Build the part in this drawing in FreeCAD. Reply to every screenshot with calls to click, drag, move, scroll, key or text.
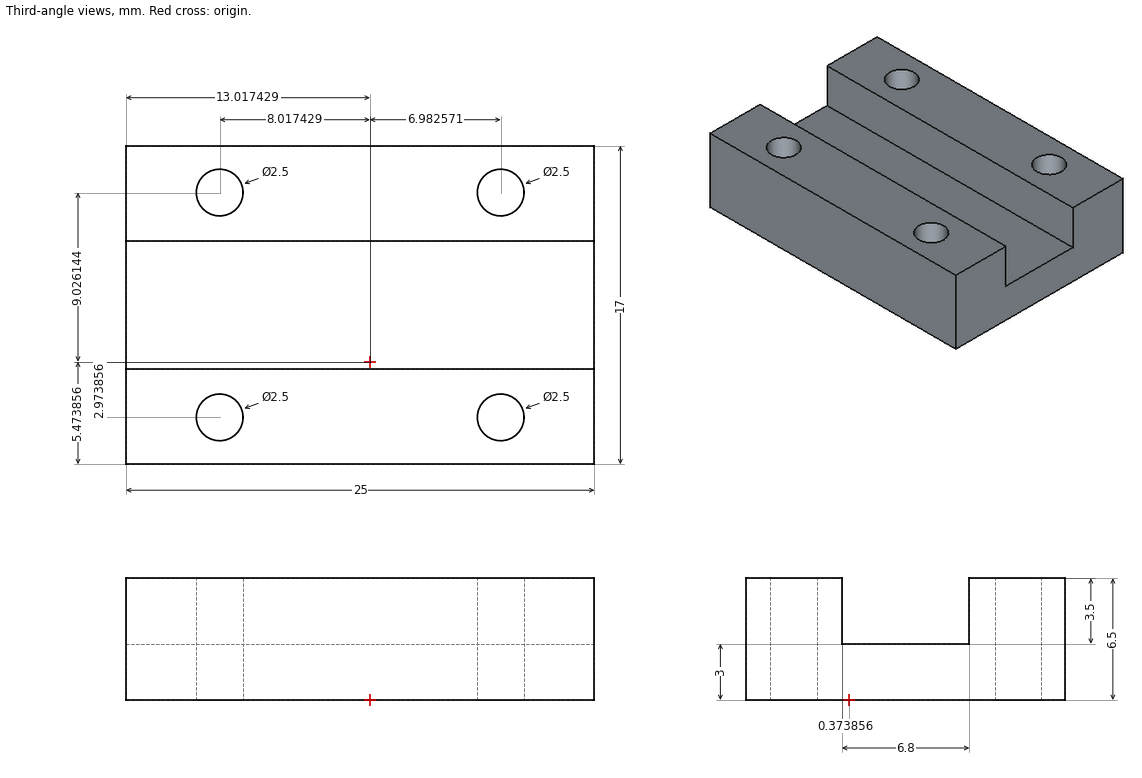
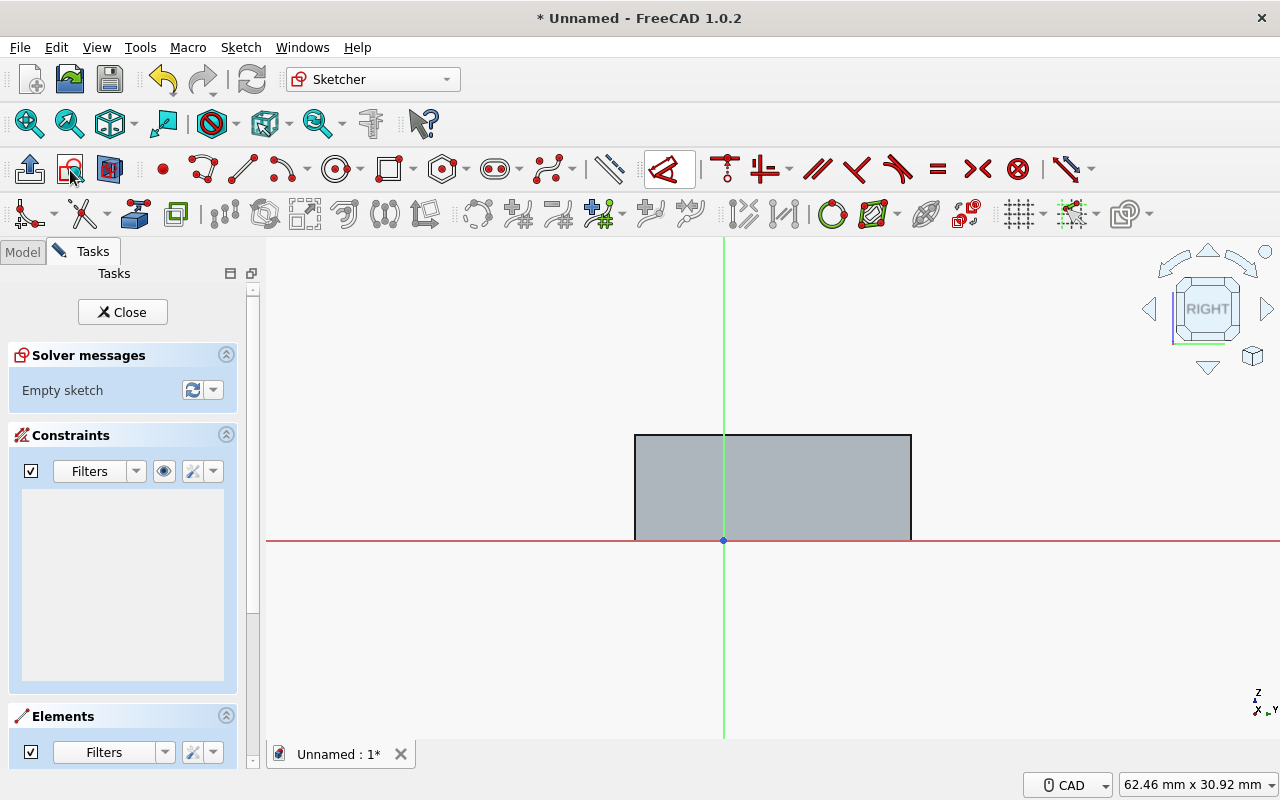
scroll(813, 488, up, 5)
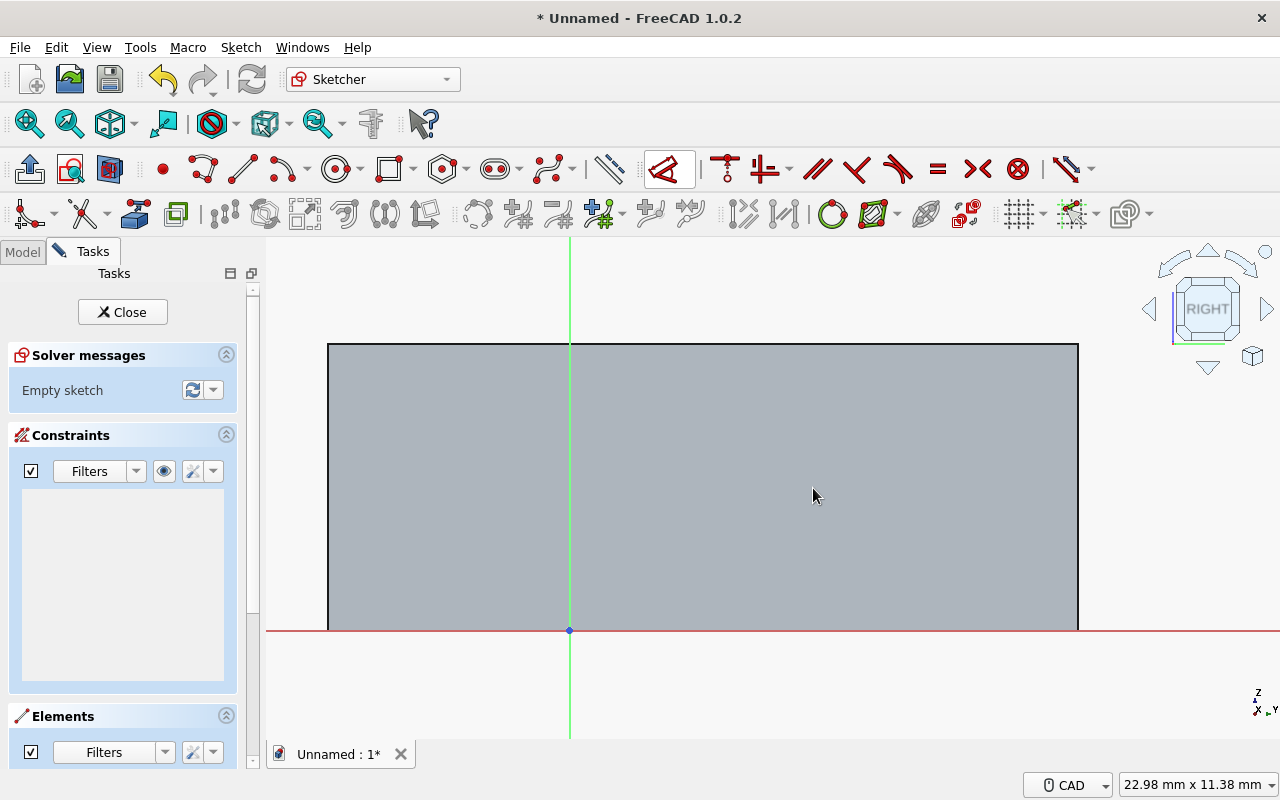
click(390, 170)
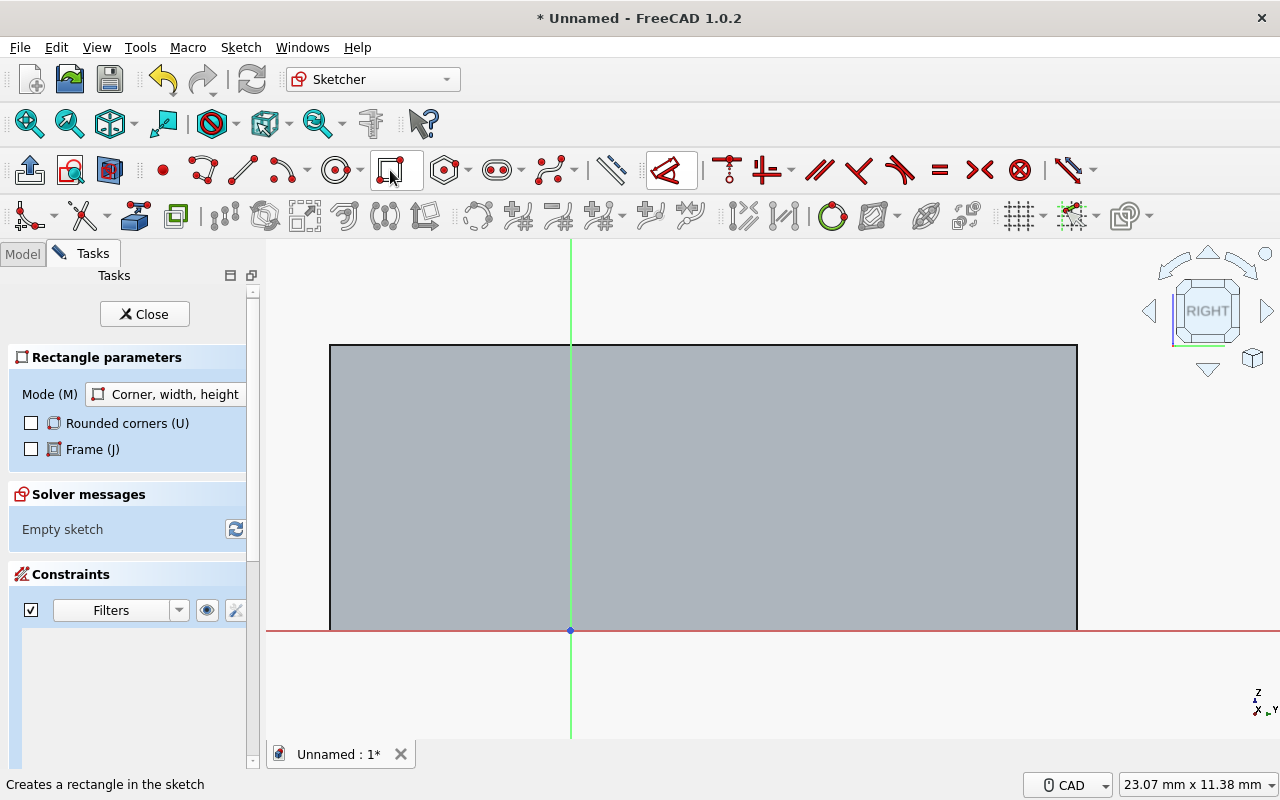
click(554, 345)
move(853, 499)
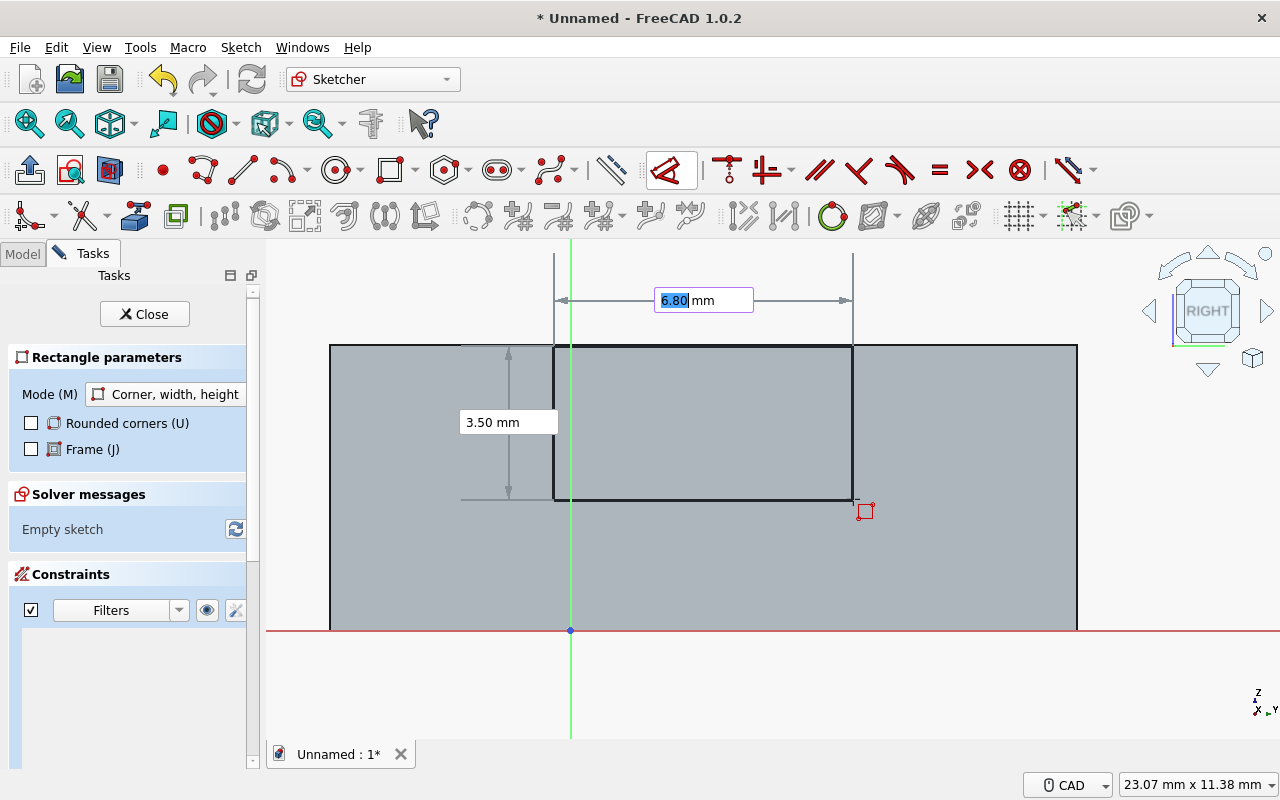
text(6.8)
key(Tab)
text(3.5)
key(Return)
key(Escape)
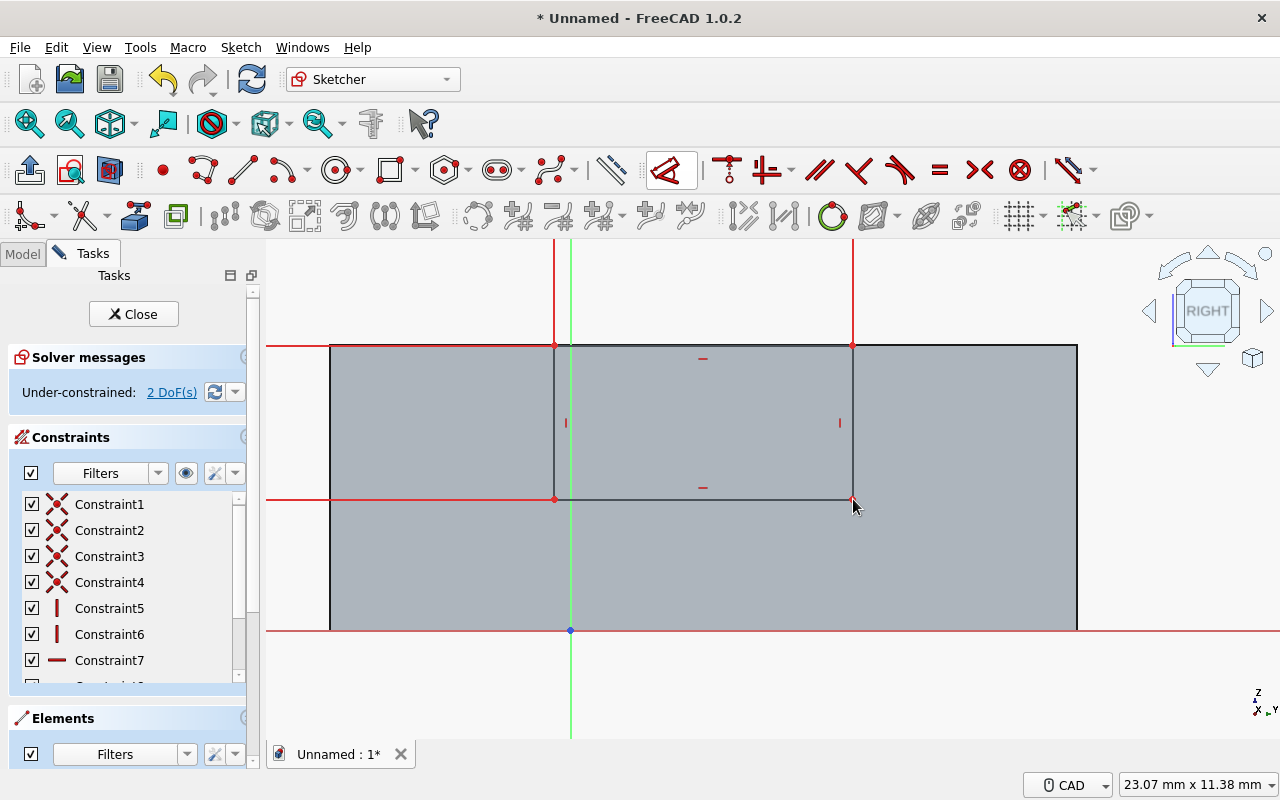
click(666, 170)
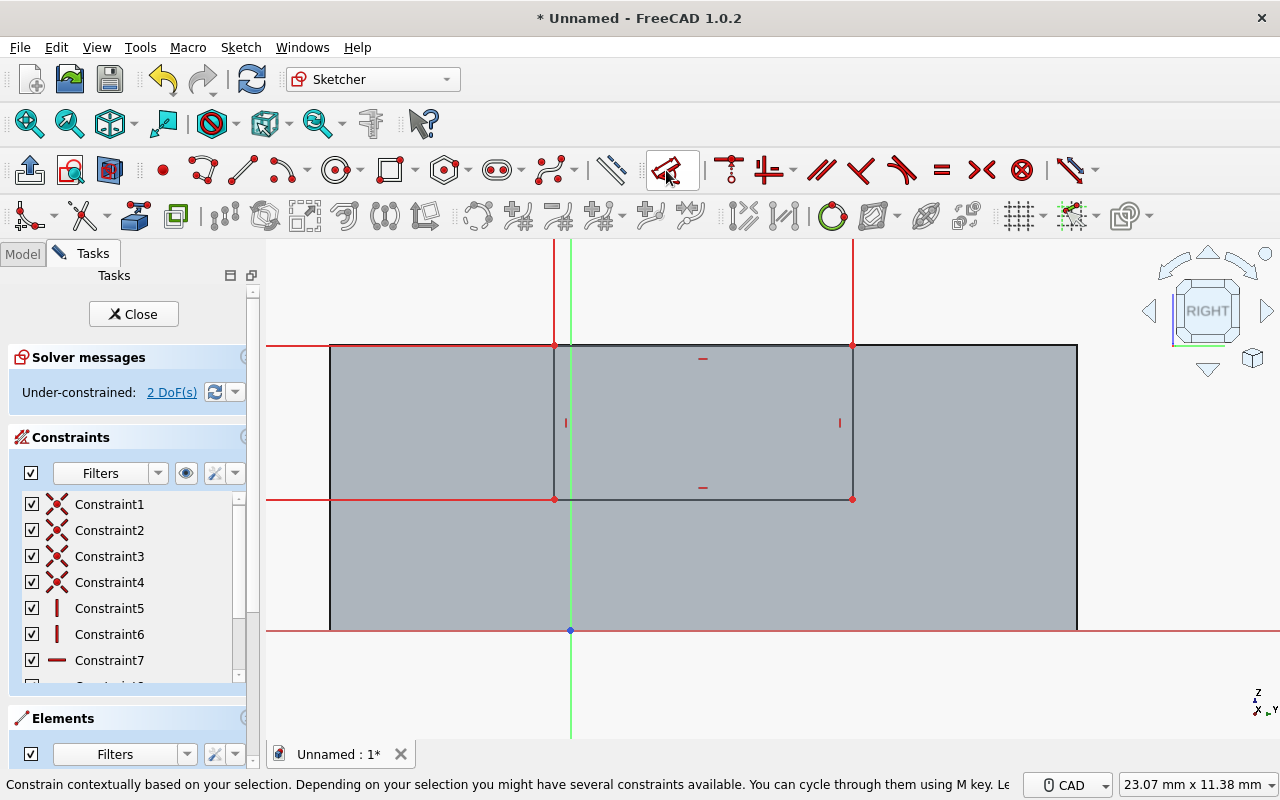
click(554, 500)
click(520, 565)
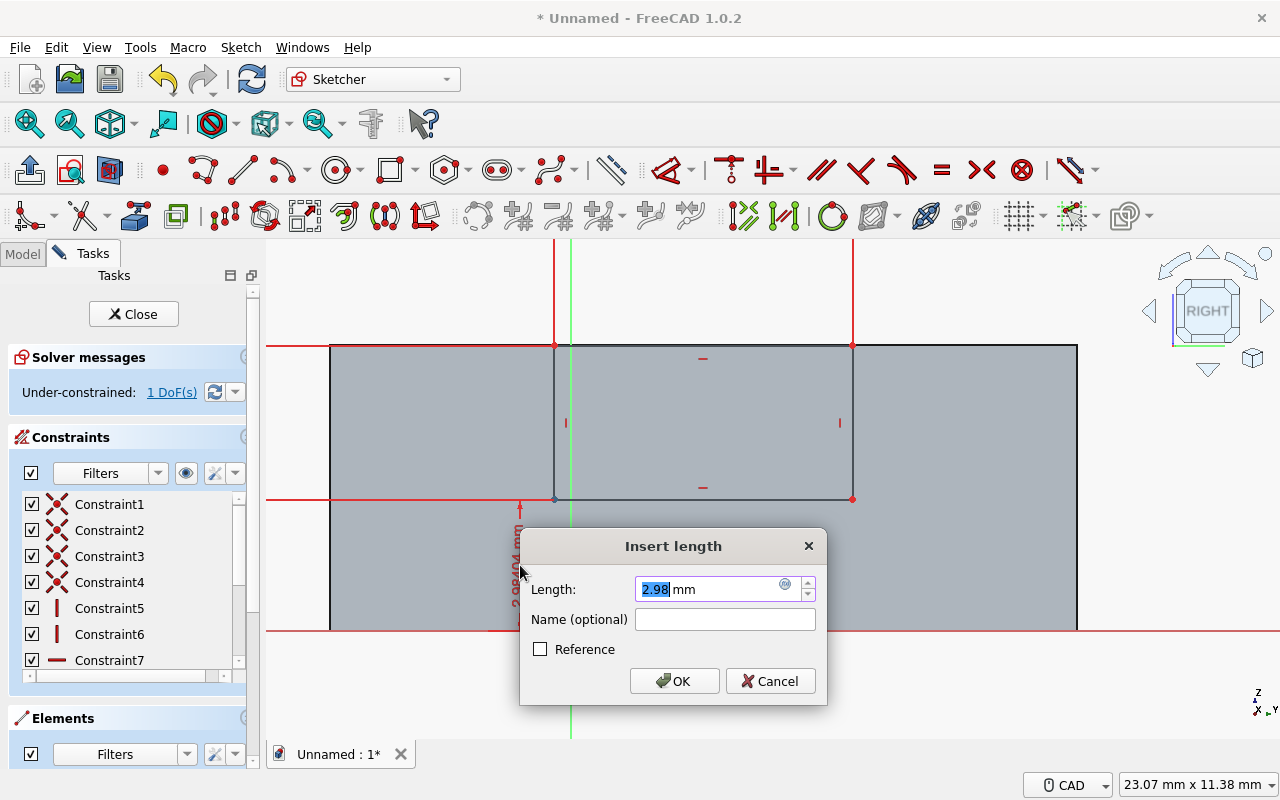
text(3)
key(Return)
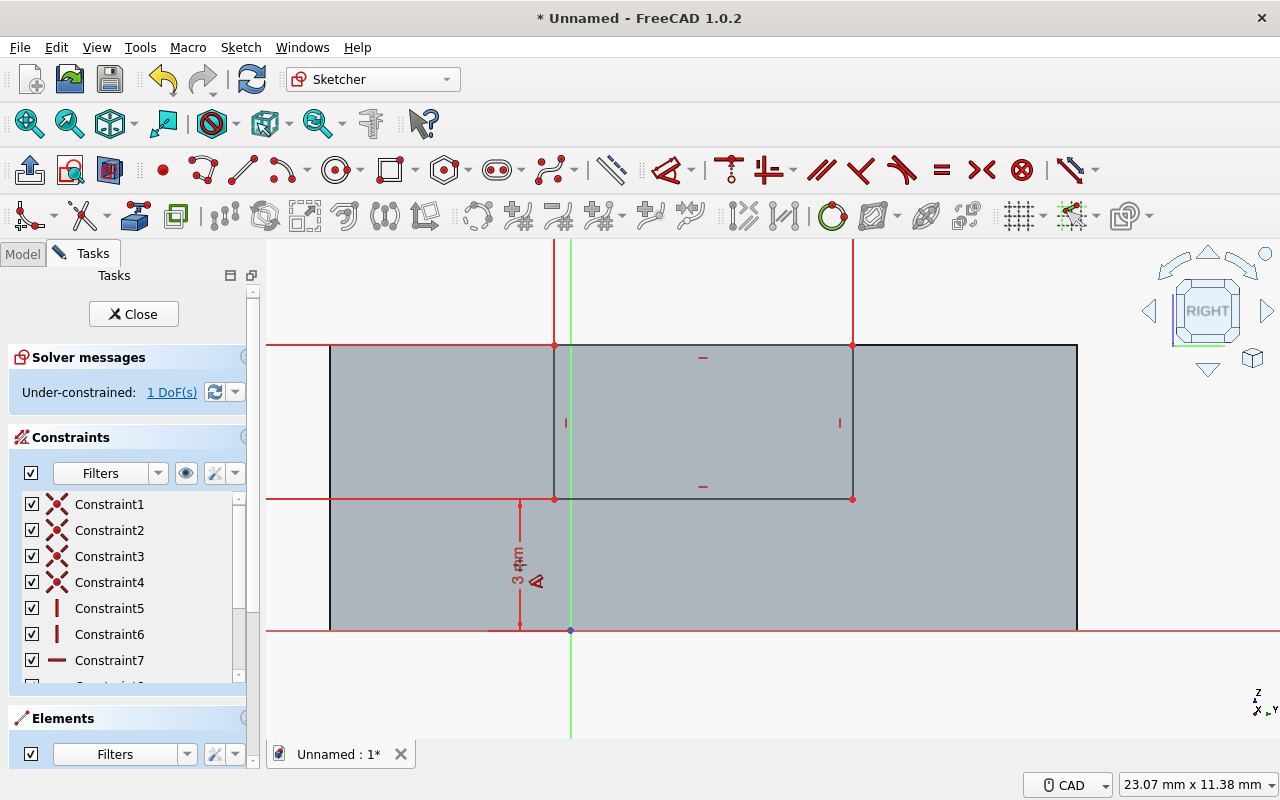
scroll(554, 345, up, 5)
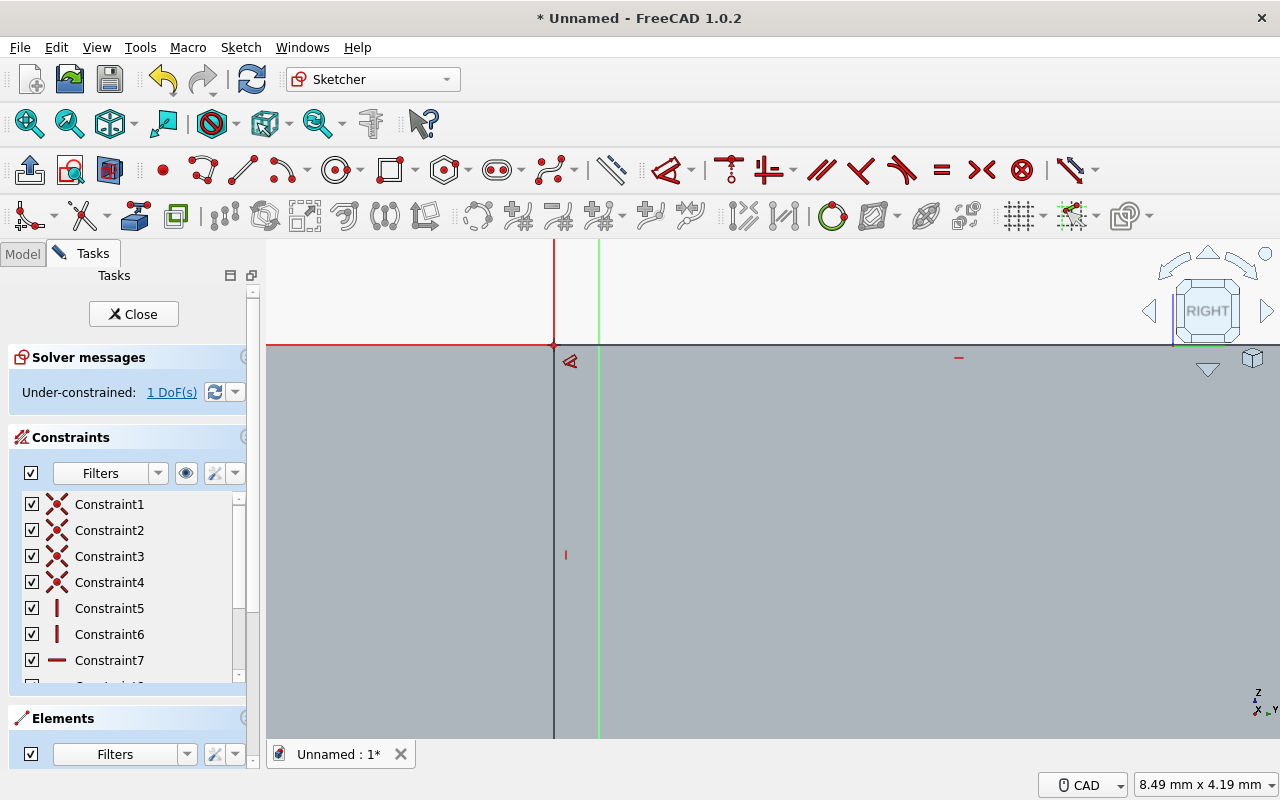
click(554, 345)
click(576, 311)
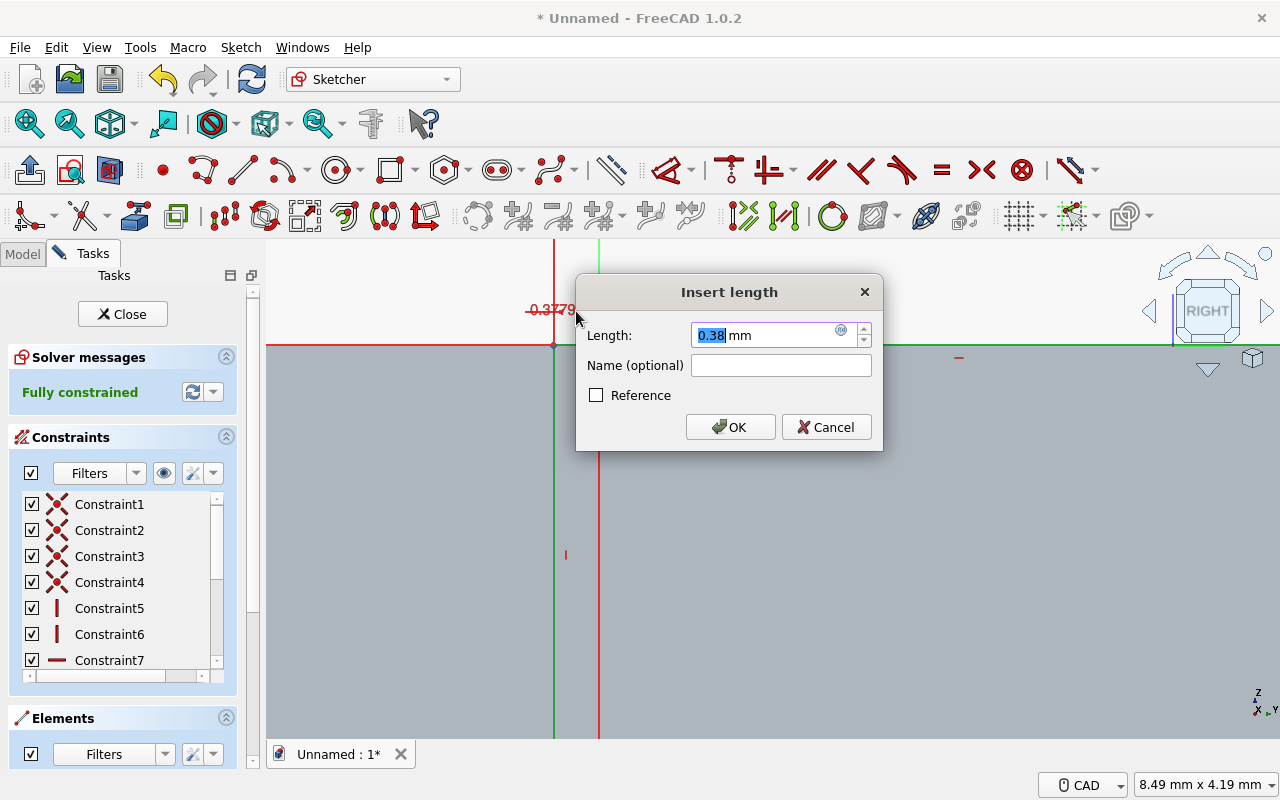
text(0.373856)
key(Return)
key(Escape)